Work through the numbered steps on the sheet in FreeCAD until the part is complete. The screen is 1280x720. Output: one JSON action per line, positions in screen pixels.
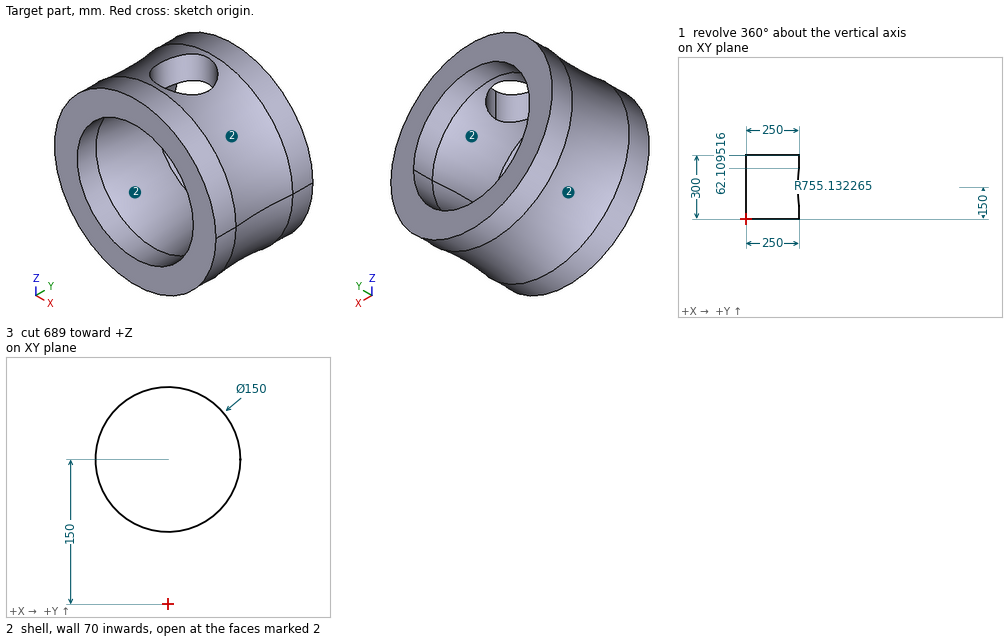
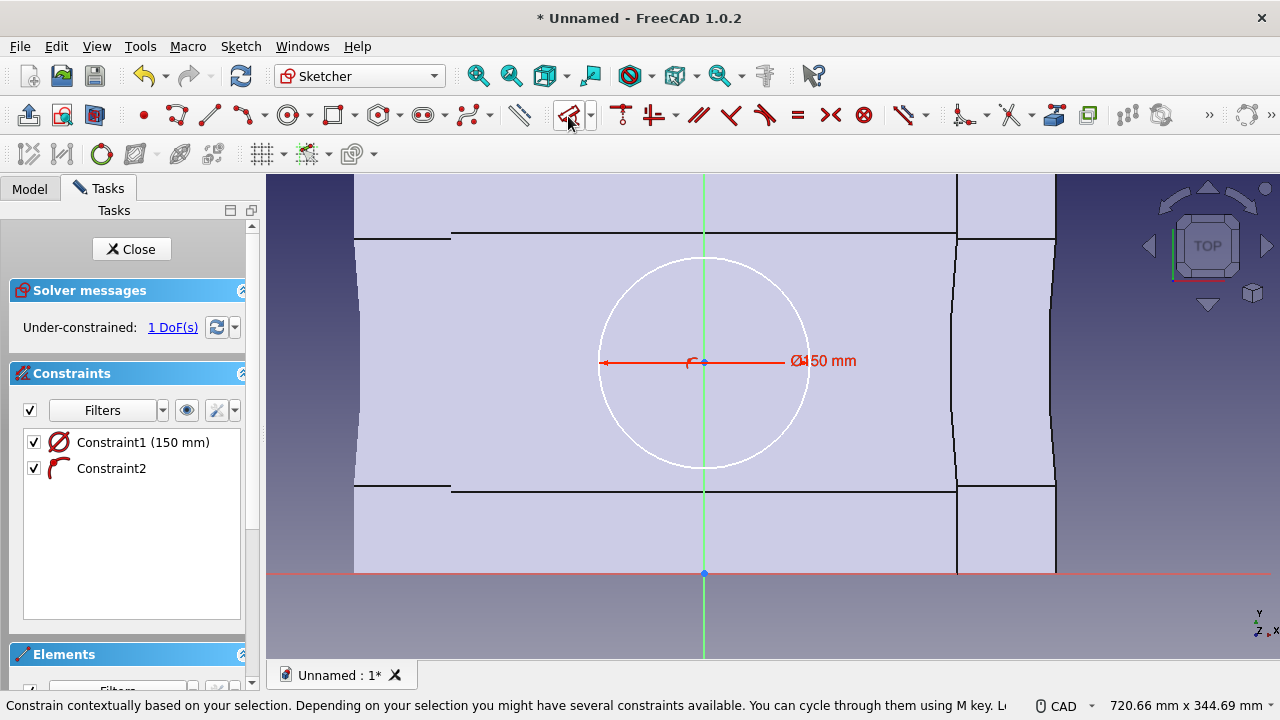
{"action": "left_click", "coordinate": [704, 363]}
{"action": "left_click", "coordinate": [738, 420]}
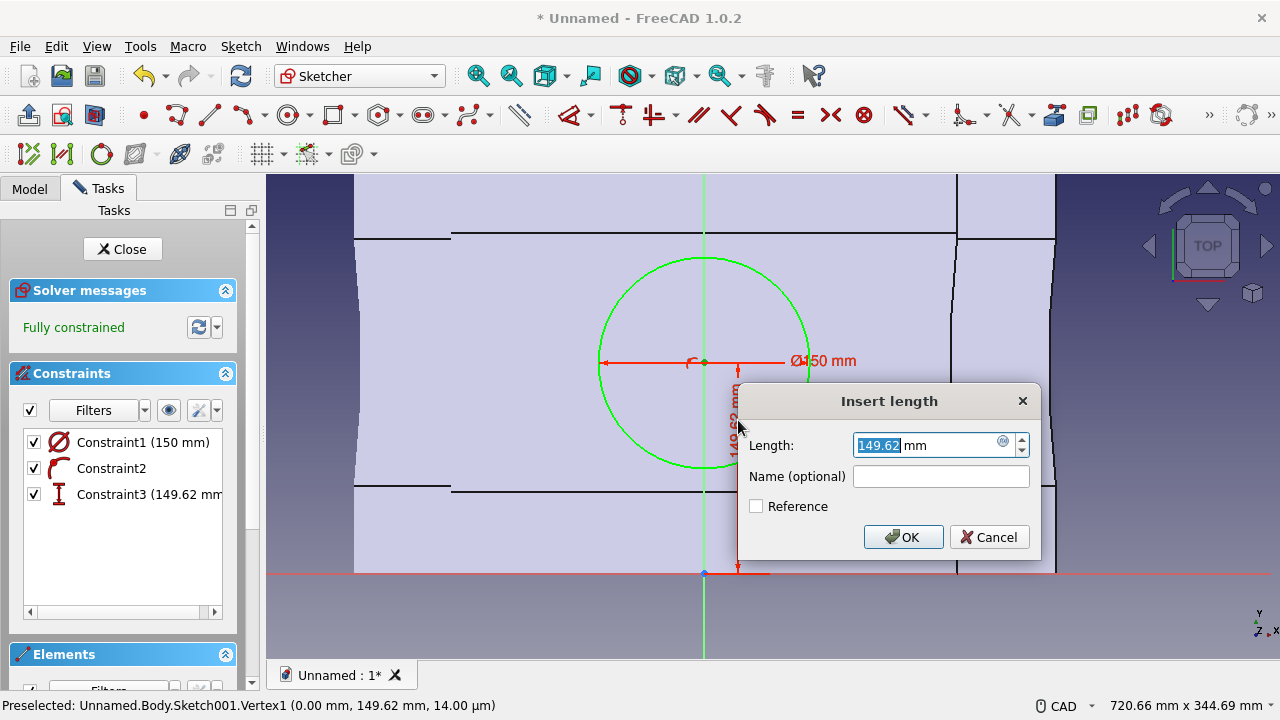
{"action": "type", "text": "150"}
{"action": "key", "text": "Return"}
{"action": "key", "text": "Escape"}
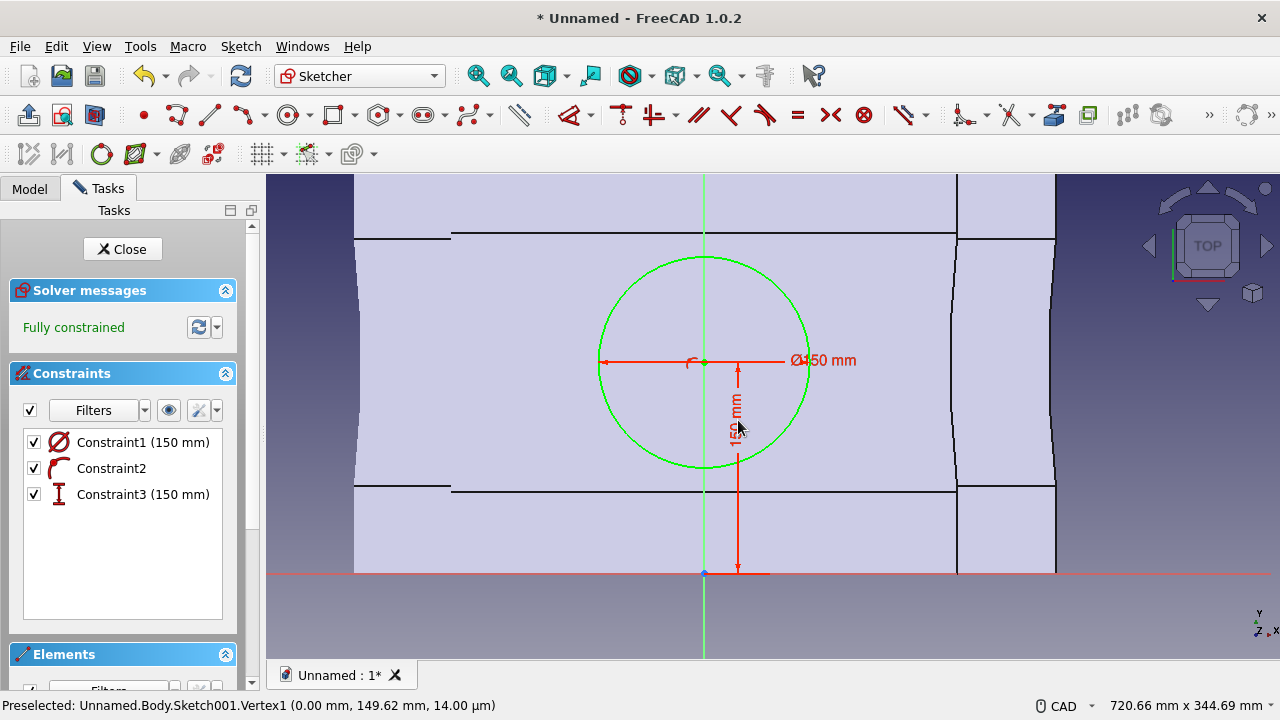
{"action": "left_click", "coordinate": [123, 249]}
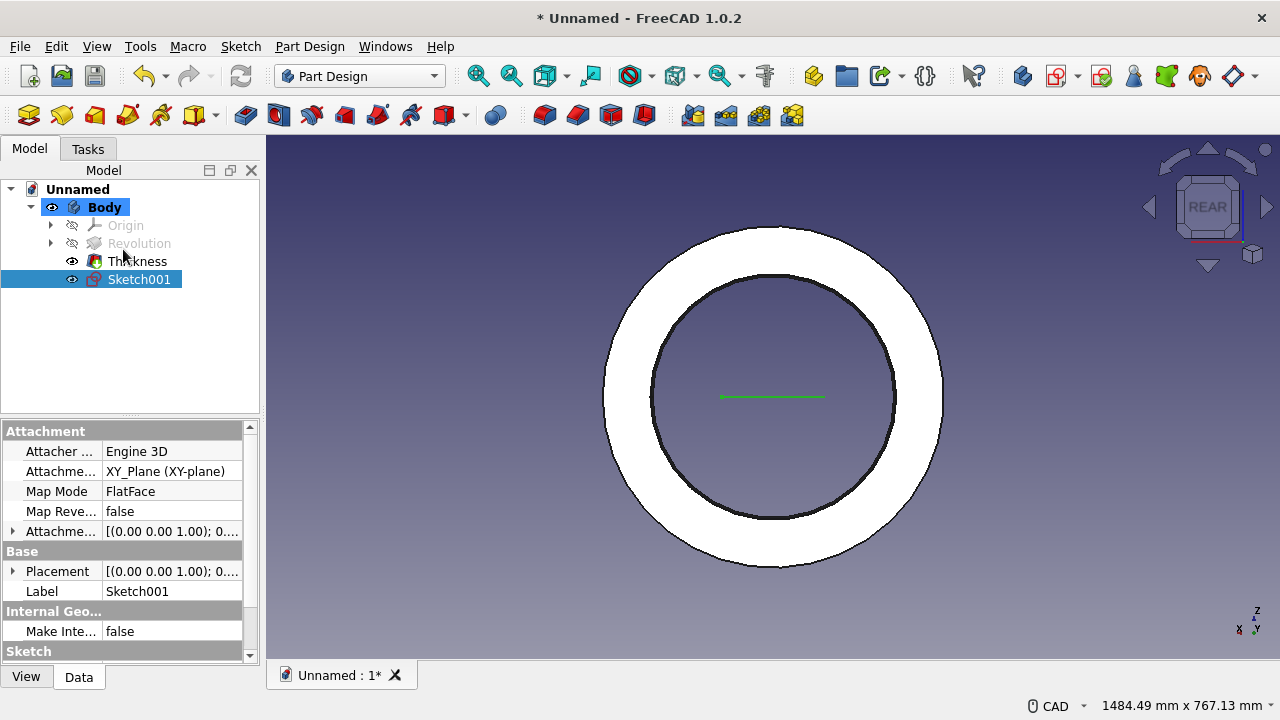
{"action": "left_click", "coordinate": [246, 116]}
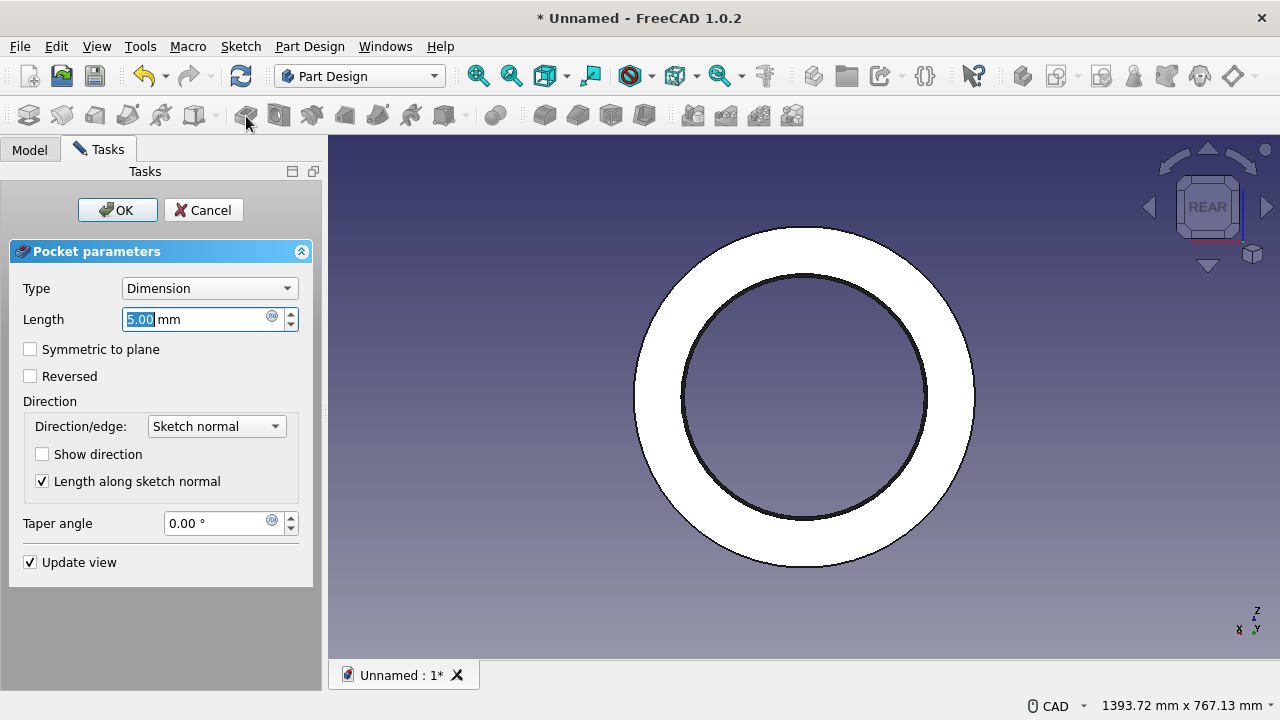
{"action": "type", "text": "689"}
{"action": "key", "text": "Tab"}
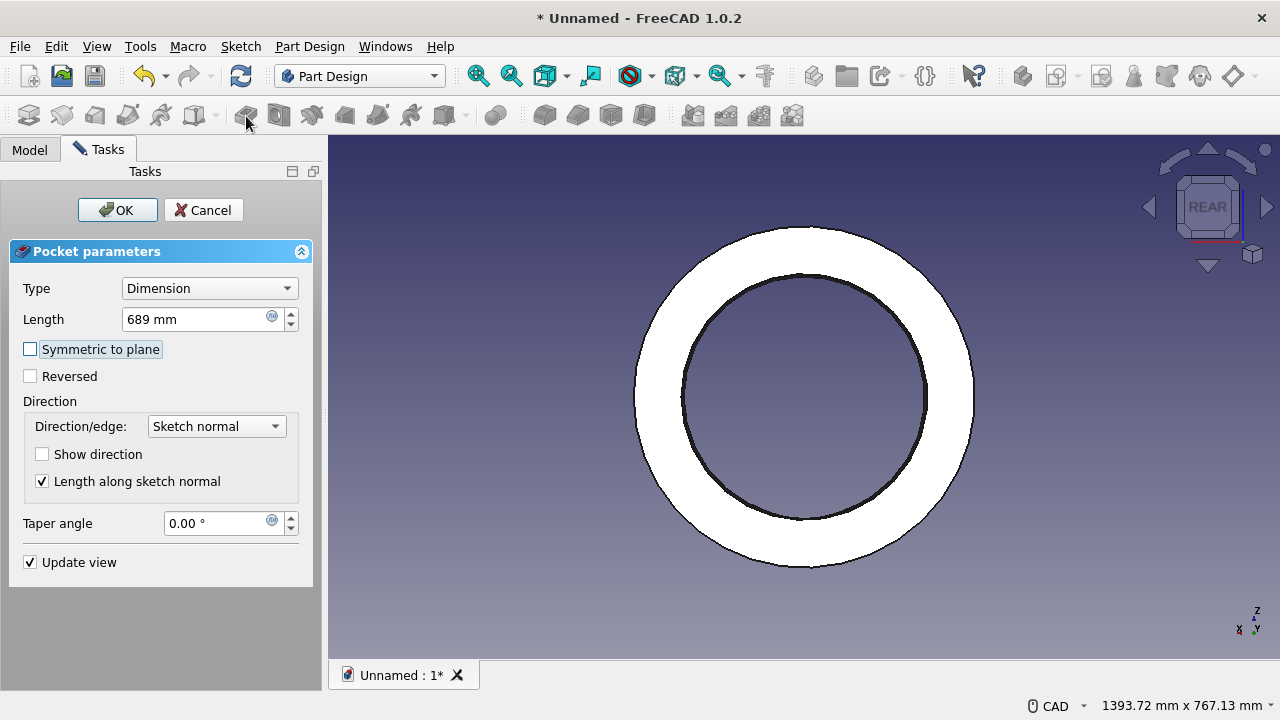
{"action": "left_click", "coordinate": [31, 376]}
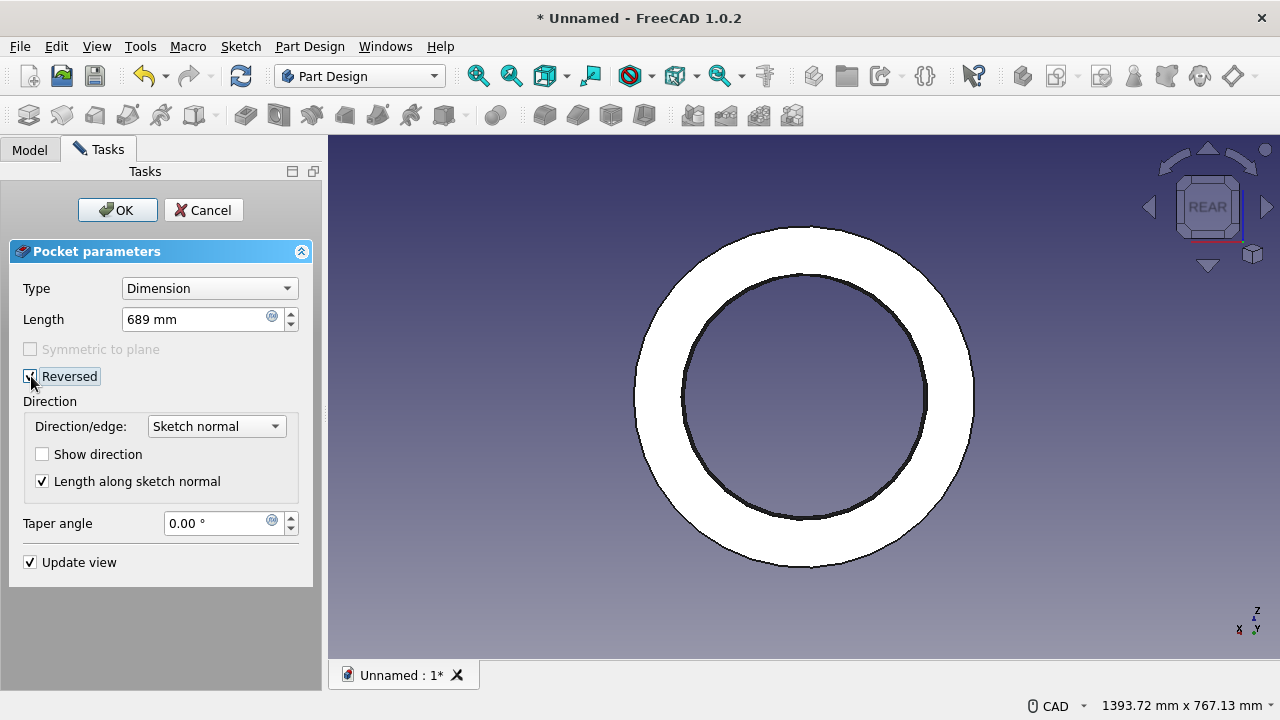
{"action": "left_click", "coordinate": [118, 210]}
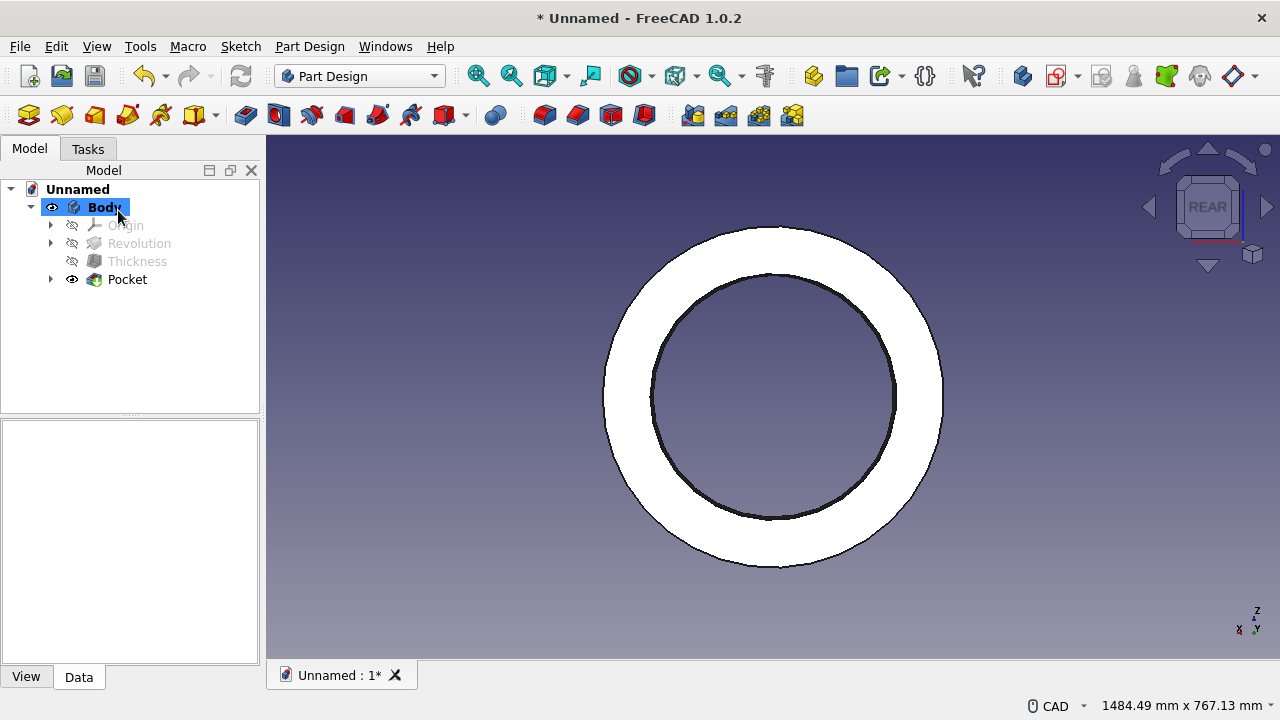
{"action": "key", "text": "0"}